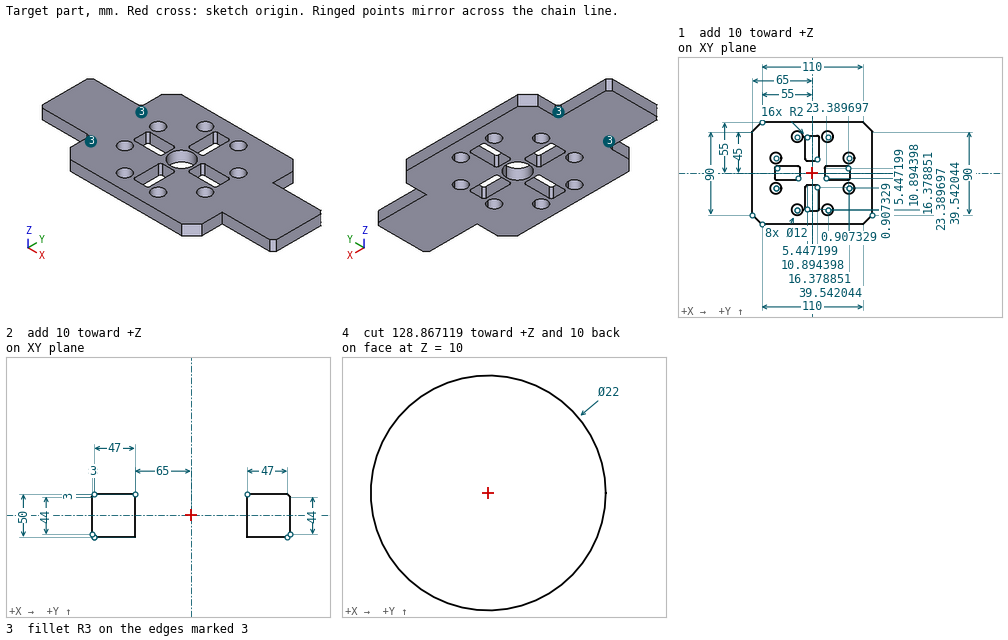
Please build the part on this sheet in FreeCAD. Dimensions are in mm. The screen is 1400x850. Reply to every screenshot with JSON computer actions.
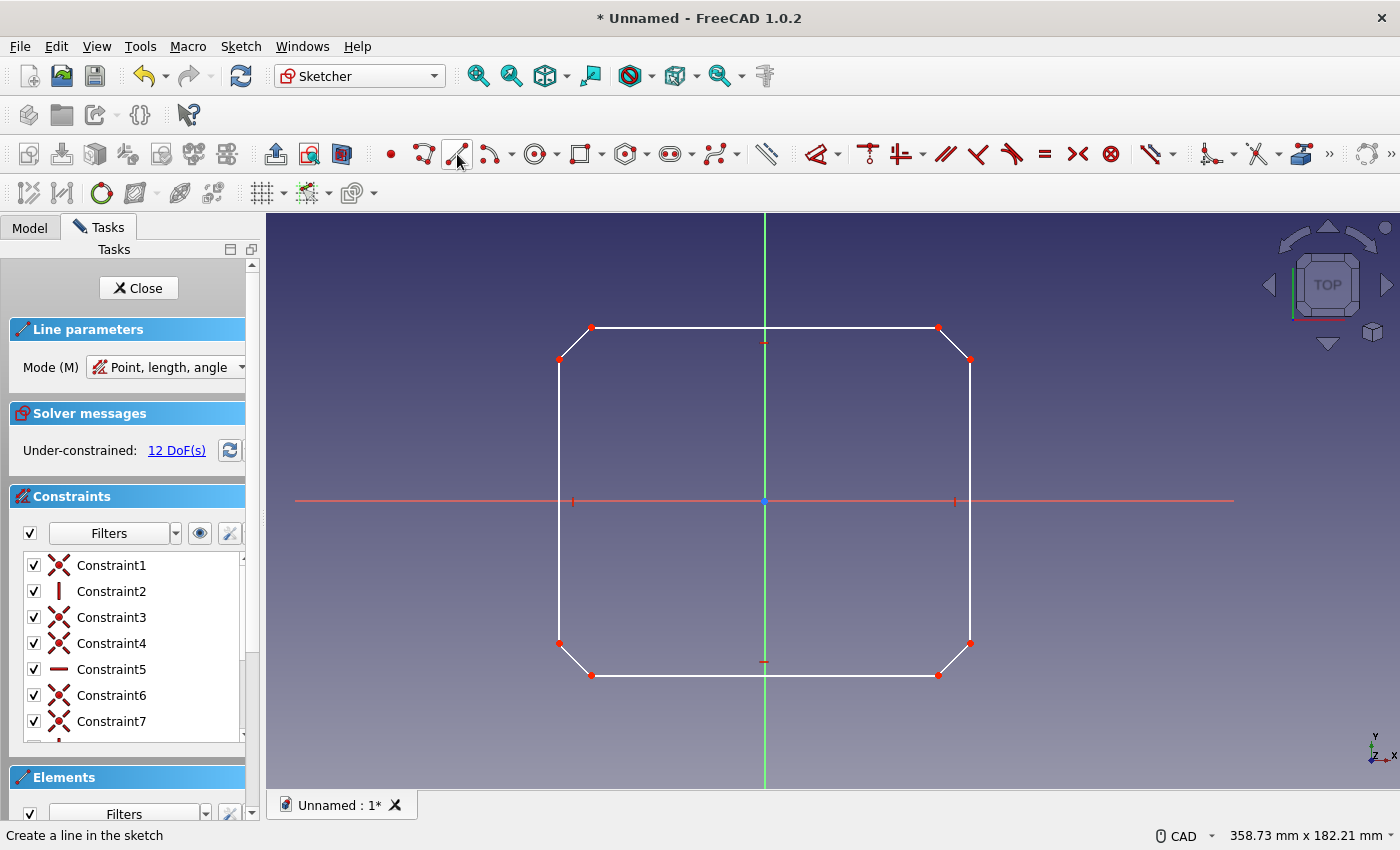
{"action": "left_click", "coordinate": [747, 543]}
{"action": "left_click", "coordinate": [782, 543]}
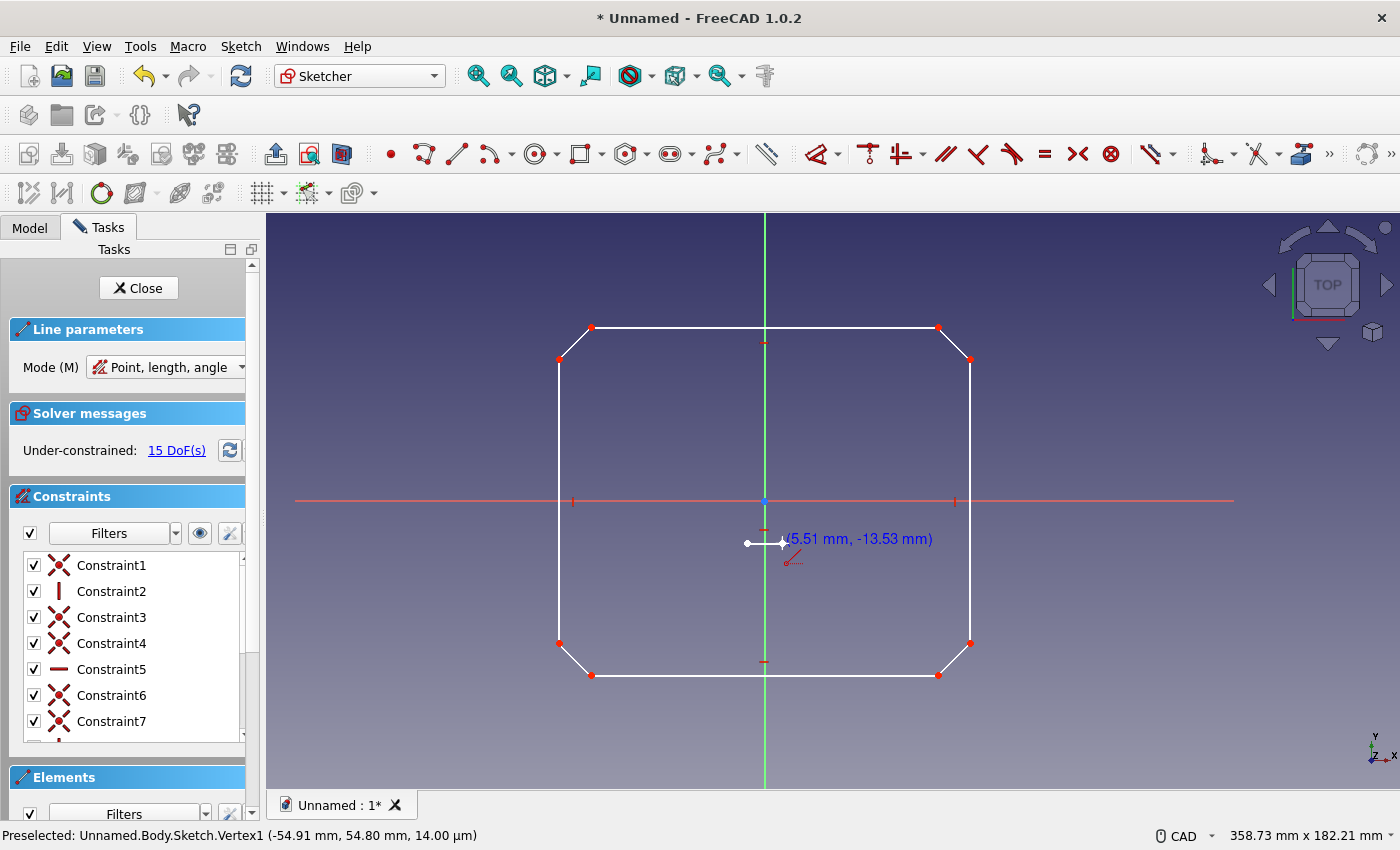
{"action": "scroll", "coordinate": [788, 549], "scroll_direction": "up", "scroll_amount": 3}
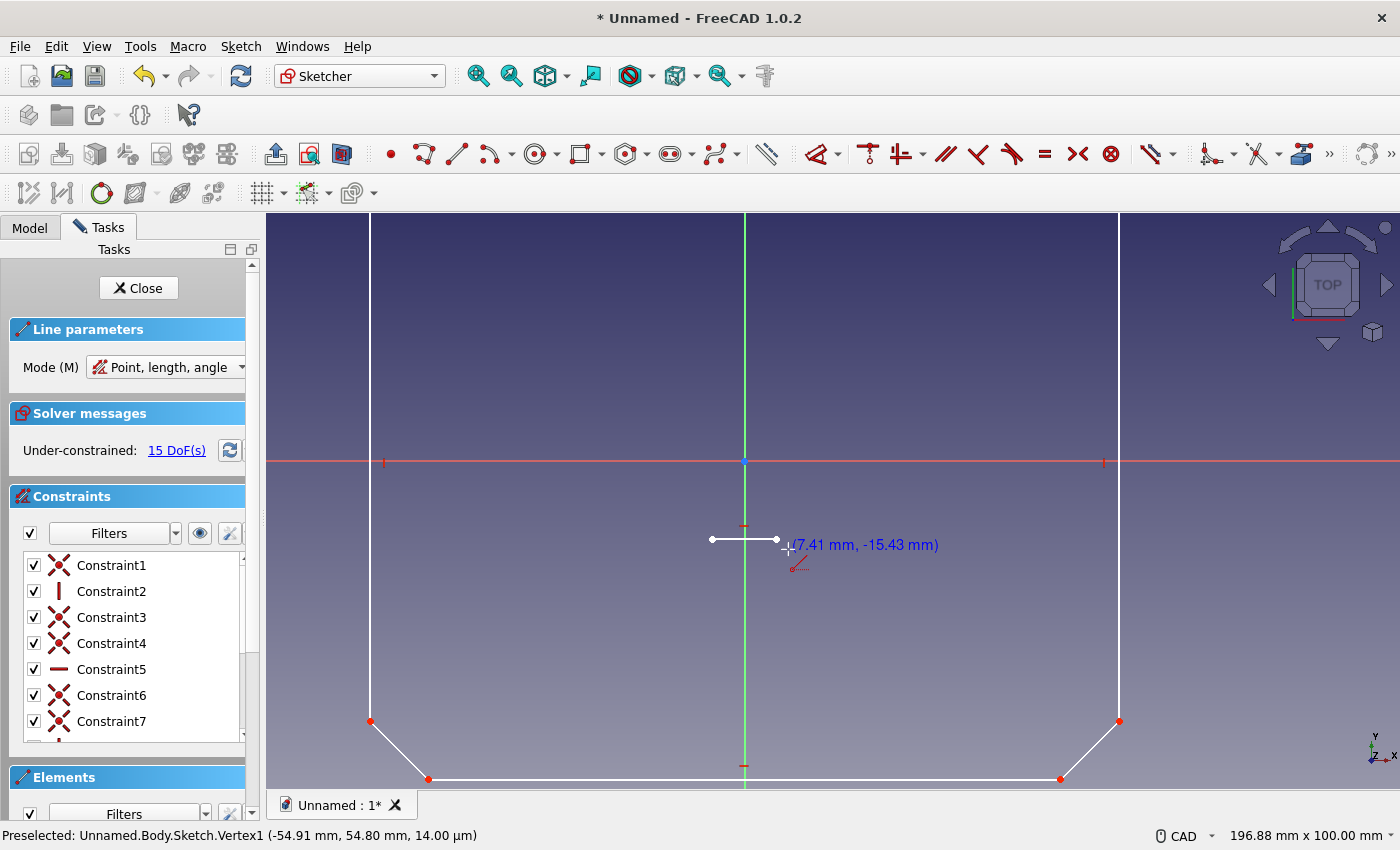
{"action": "left_click", "coordinate": [788, 549]}
{"action": "left_click", "coordinate": [788, 684]}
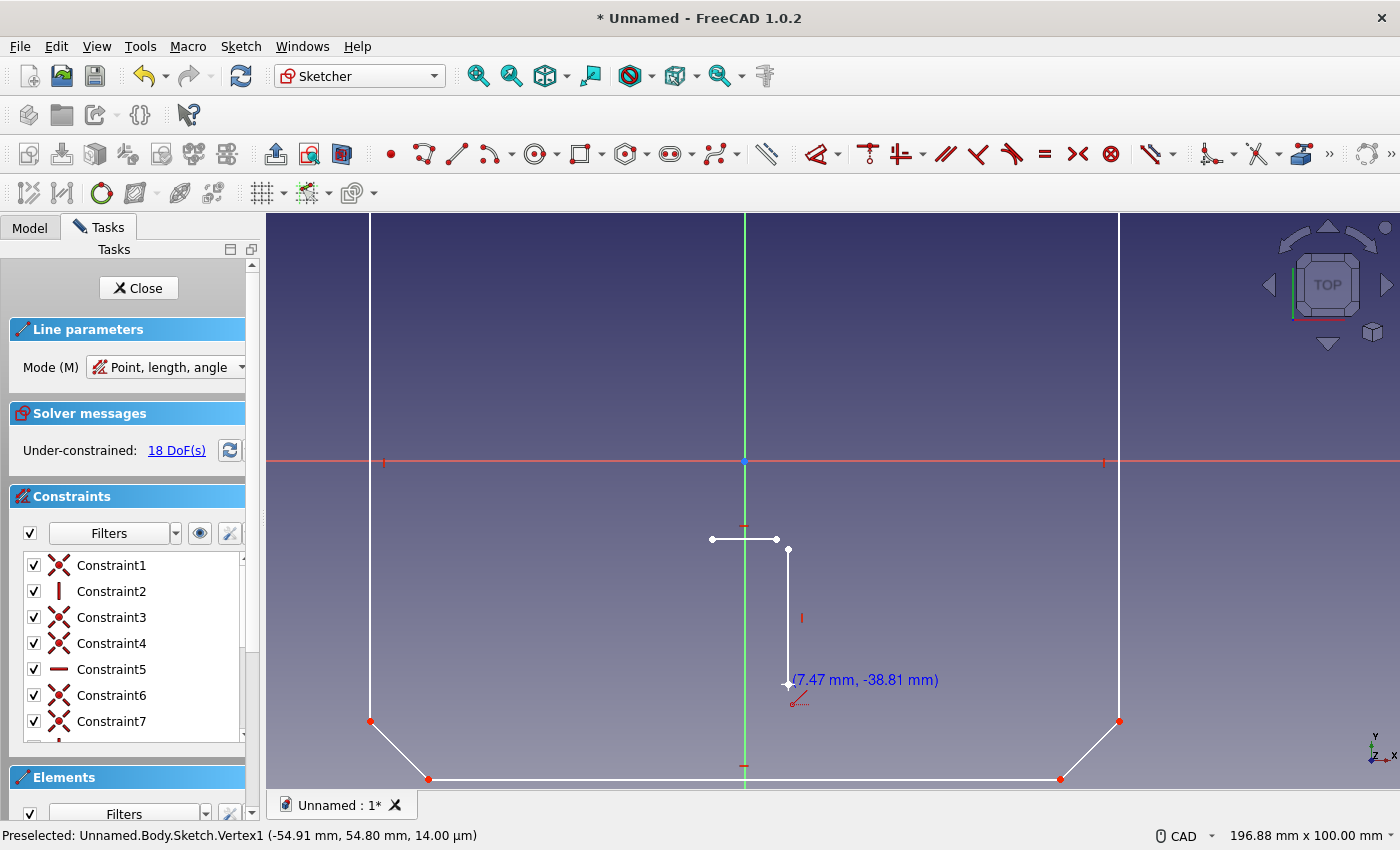
{"action": "left_click", "coordinate": [776, 696]}
{"action": "left_click", "coordinate": [714, 696]}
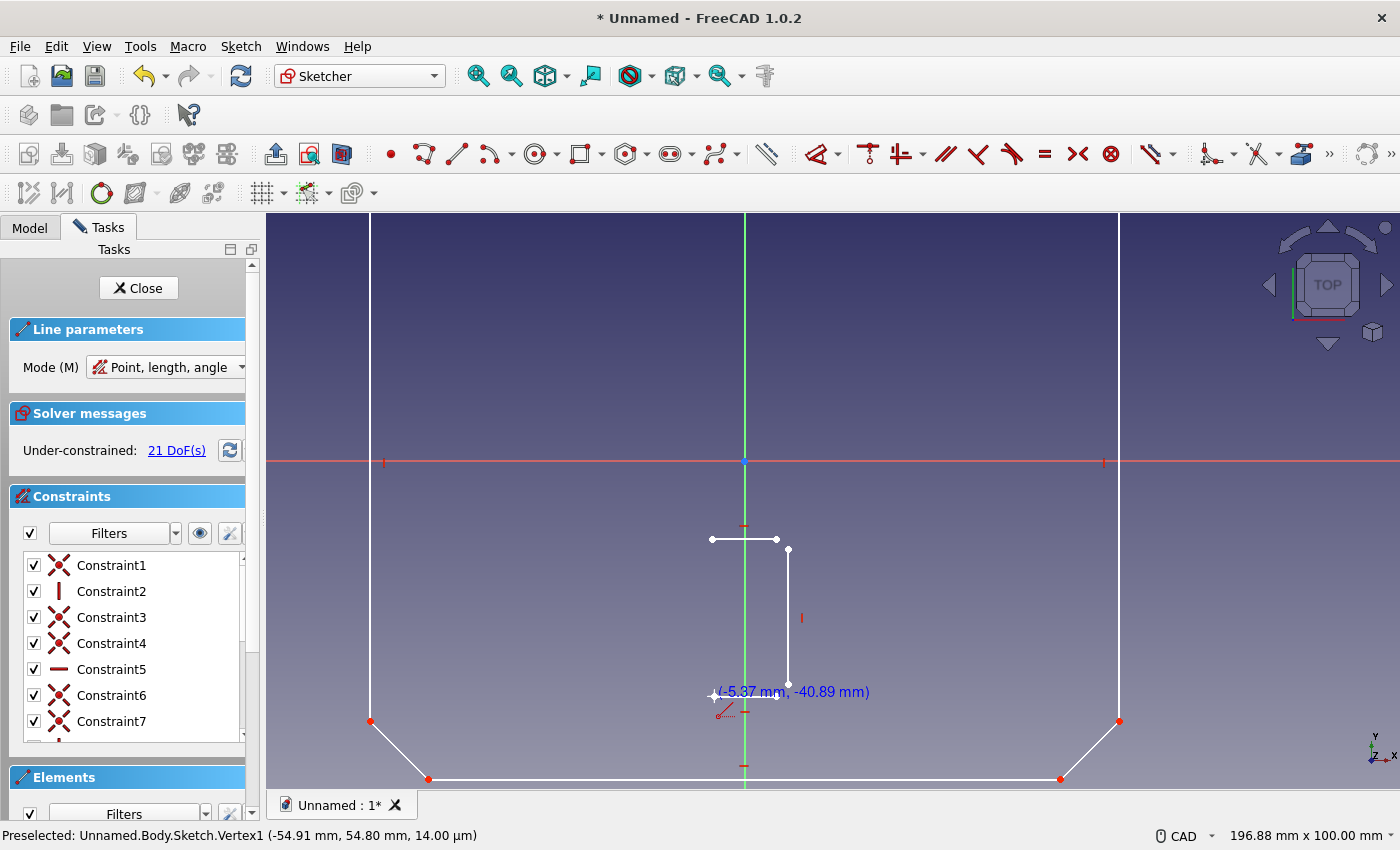
{"action": "left_click", "coordinate": [702, 684]}
{"action": "left_click", "coordinate": [702, 549]}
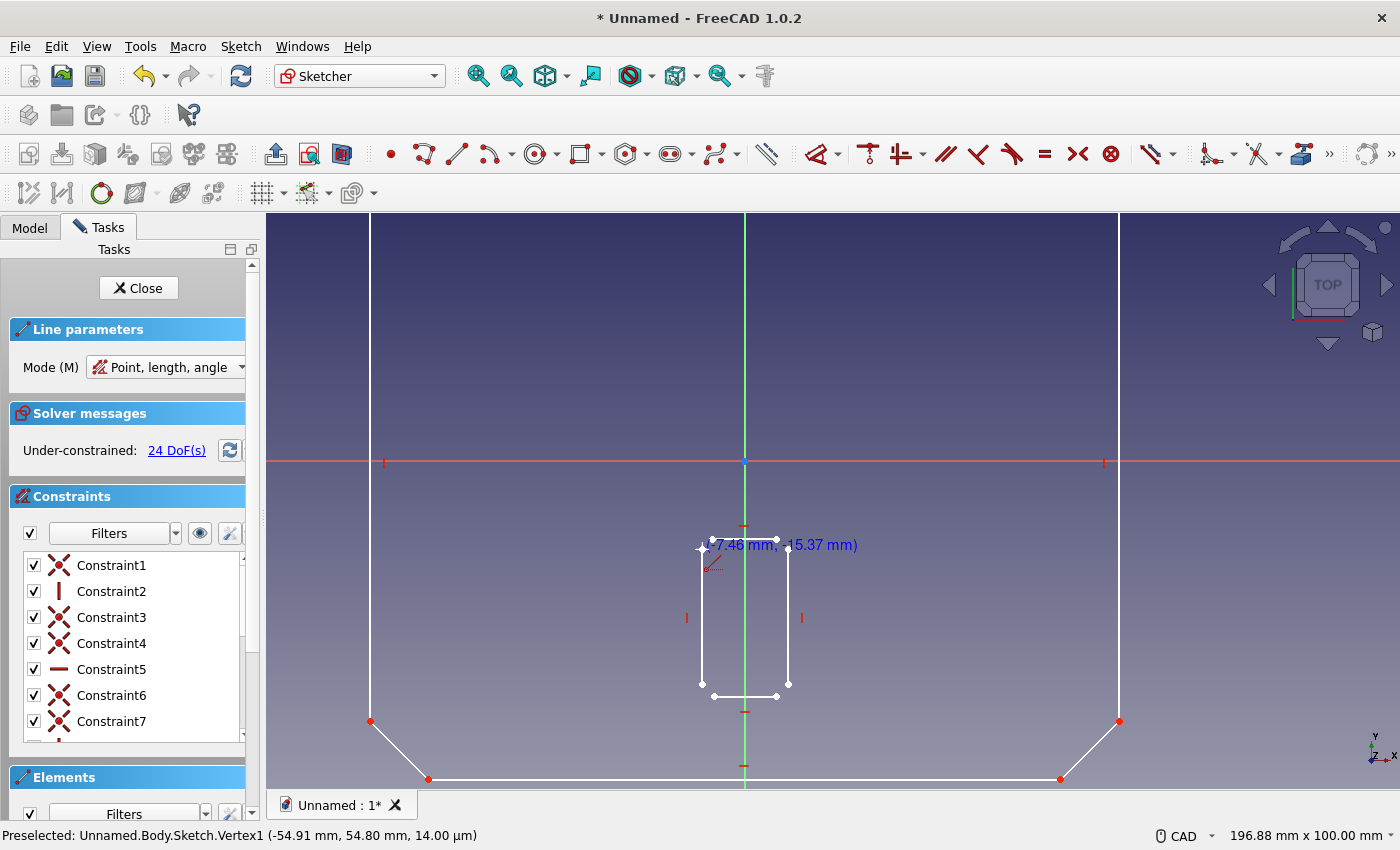
{"action": "key", "text": "g 3 a"}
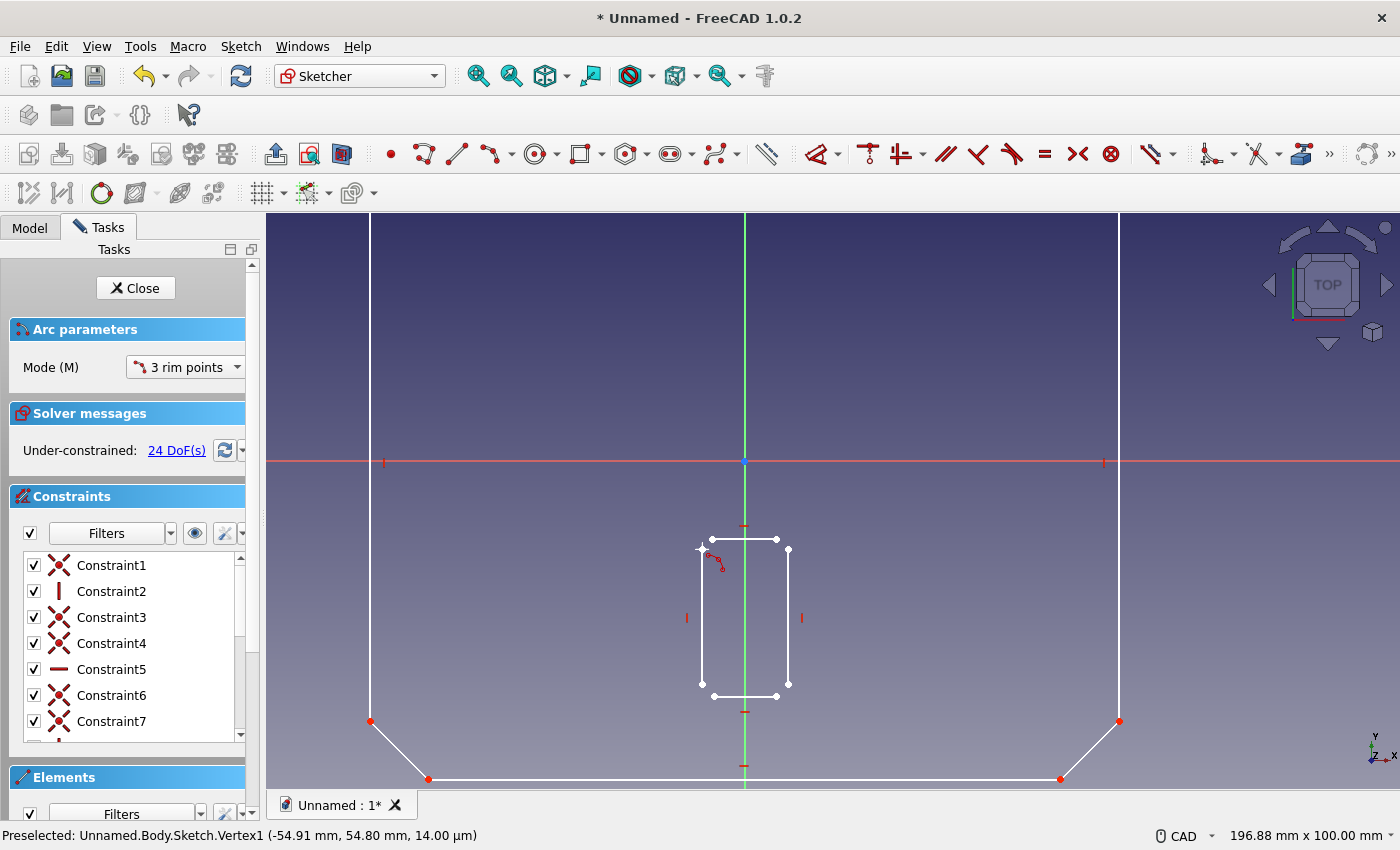
{"action": "left_click", "coordinate": [777, 539]}
{"action": "left_click", "coordinate": [788, 550]}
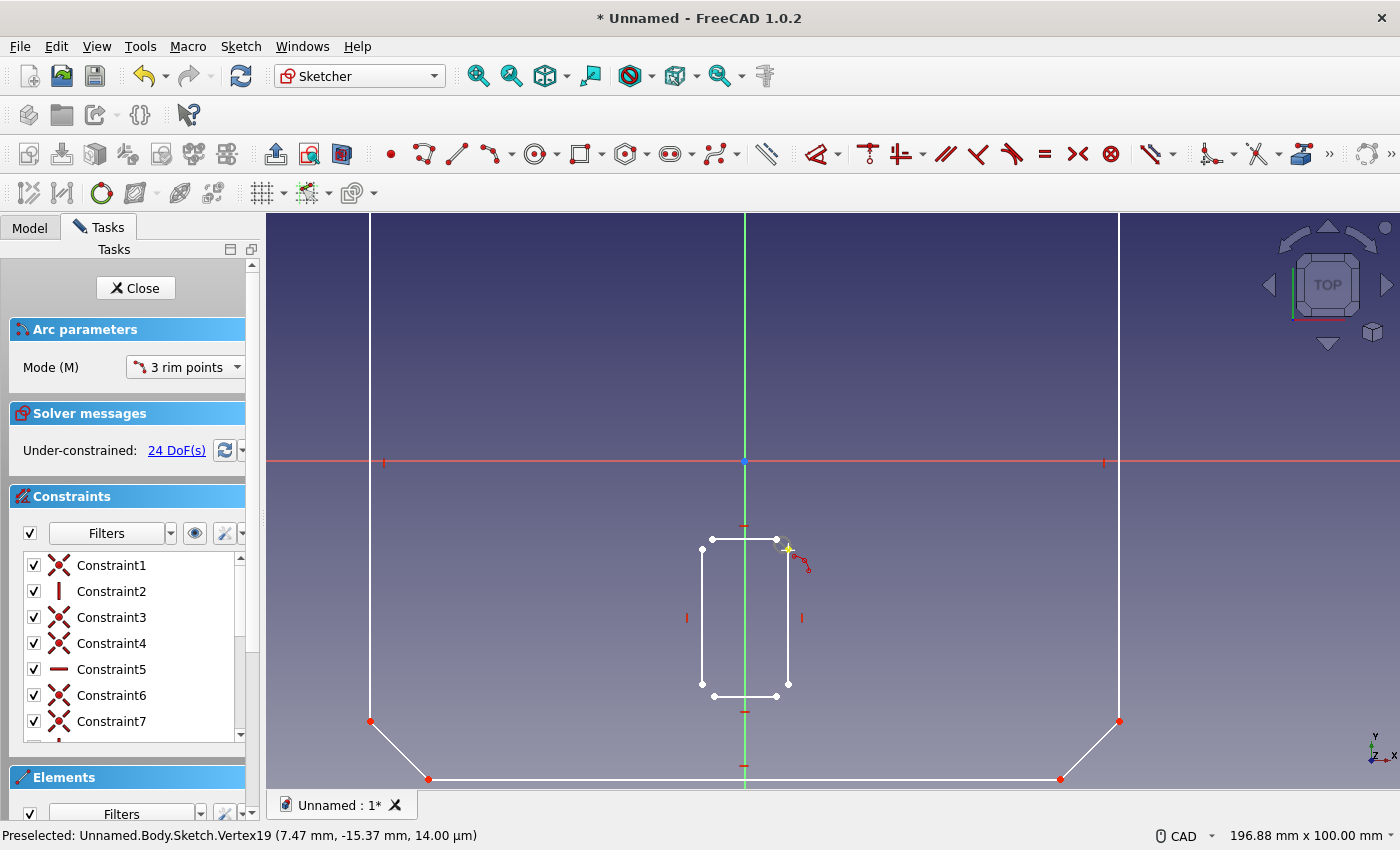
{"action": "scroll", "coordinate": [784, 541], "scroll_direction": "up", "scroll_amount": 8}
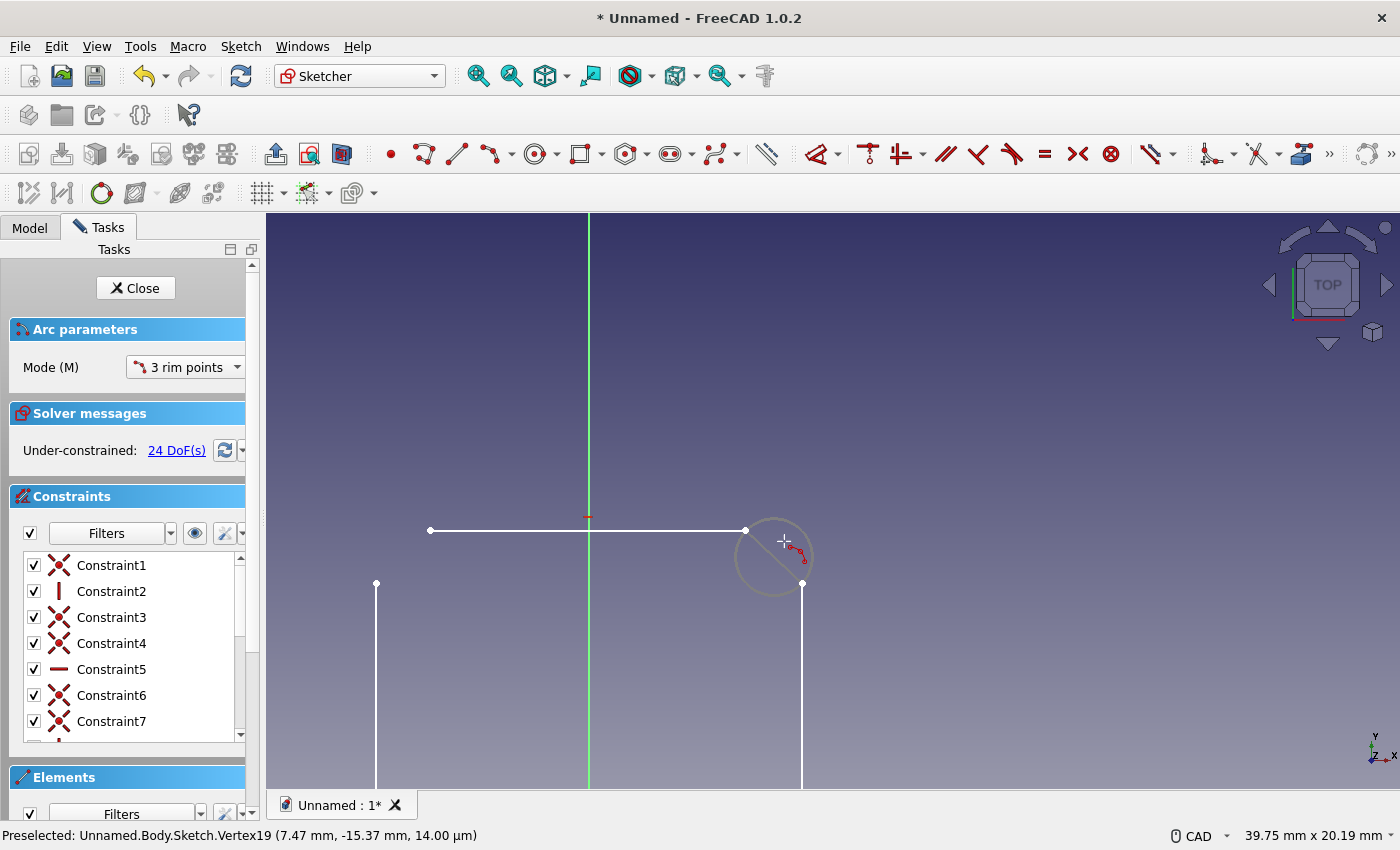
{"action": "left_click", "coordinate": [785, 539]}